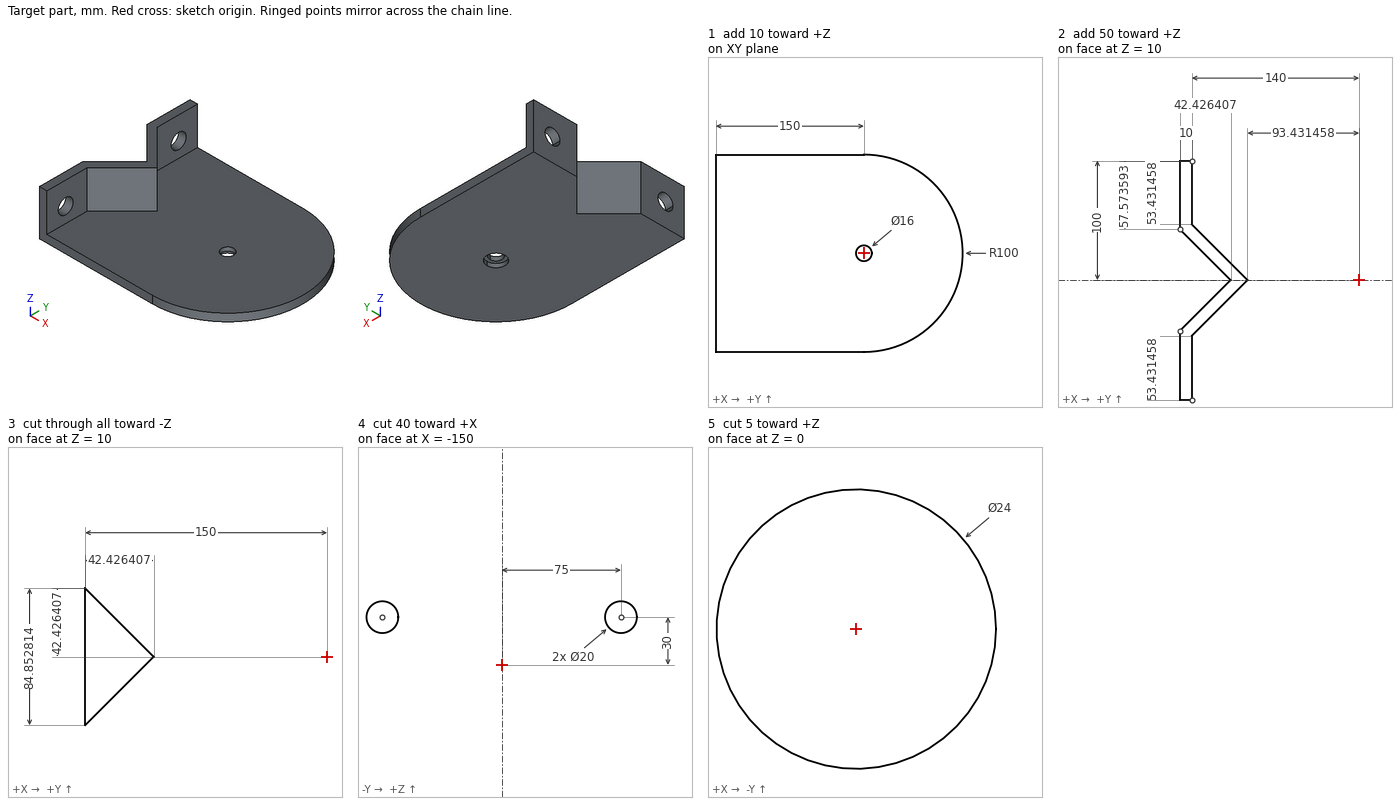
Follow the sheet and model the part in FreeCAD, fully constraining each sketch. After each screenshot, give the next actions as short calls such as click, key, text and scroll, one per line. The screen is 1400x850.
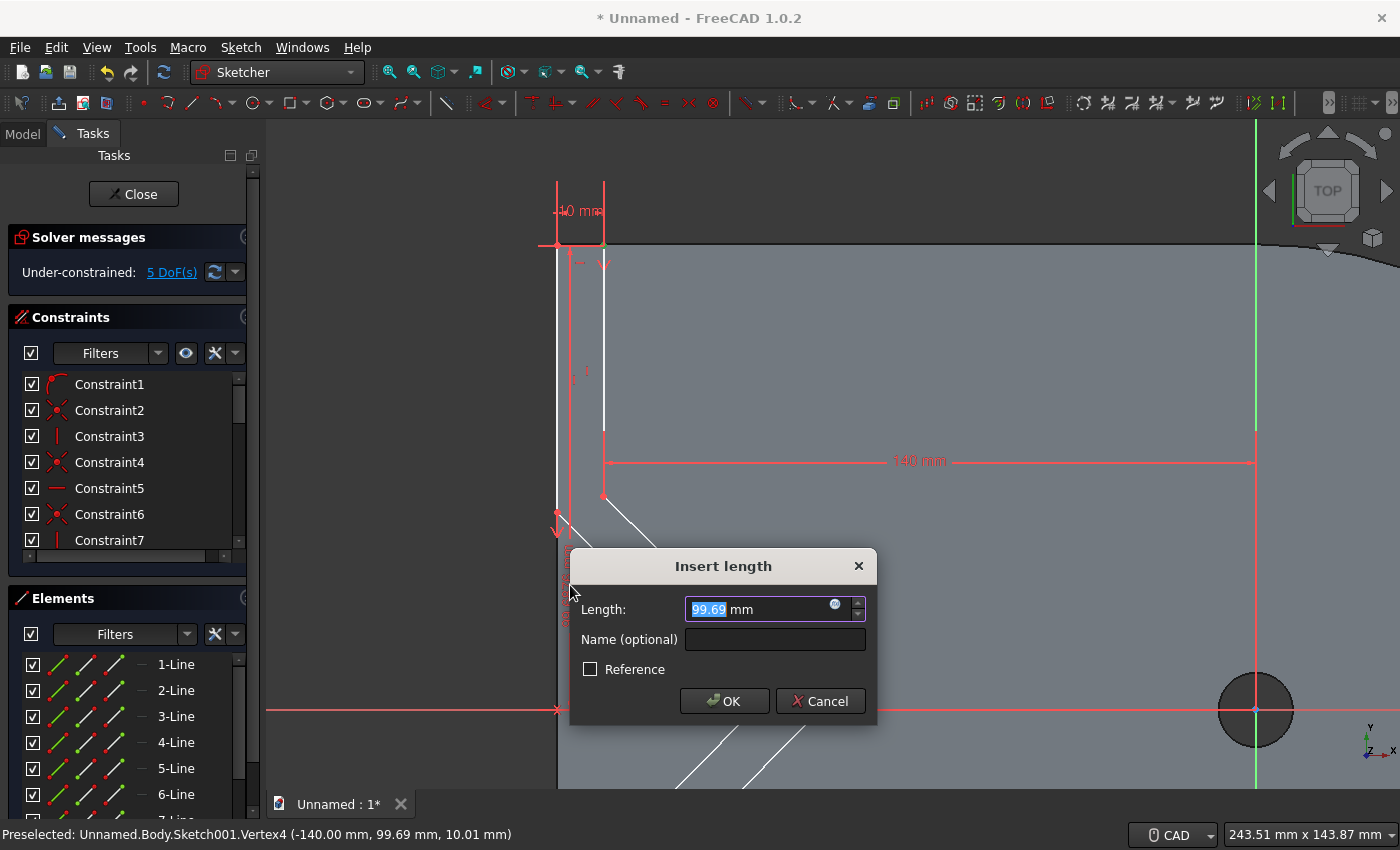
text(100)
key(Return)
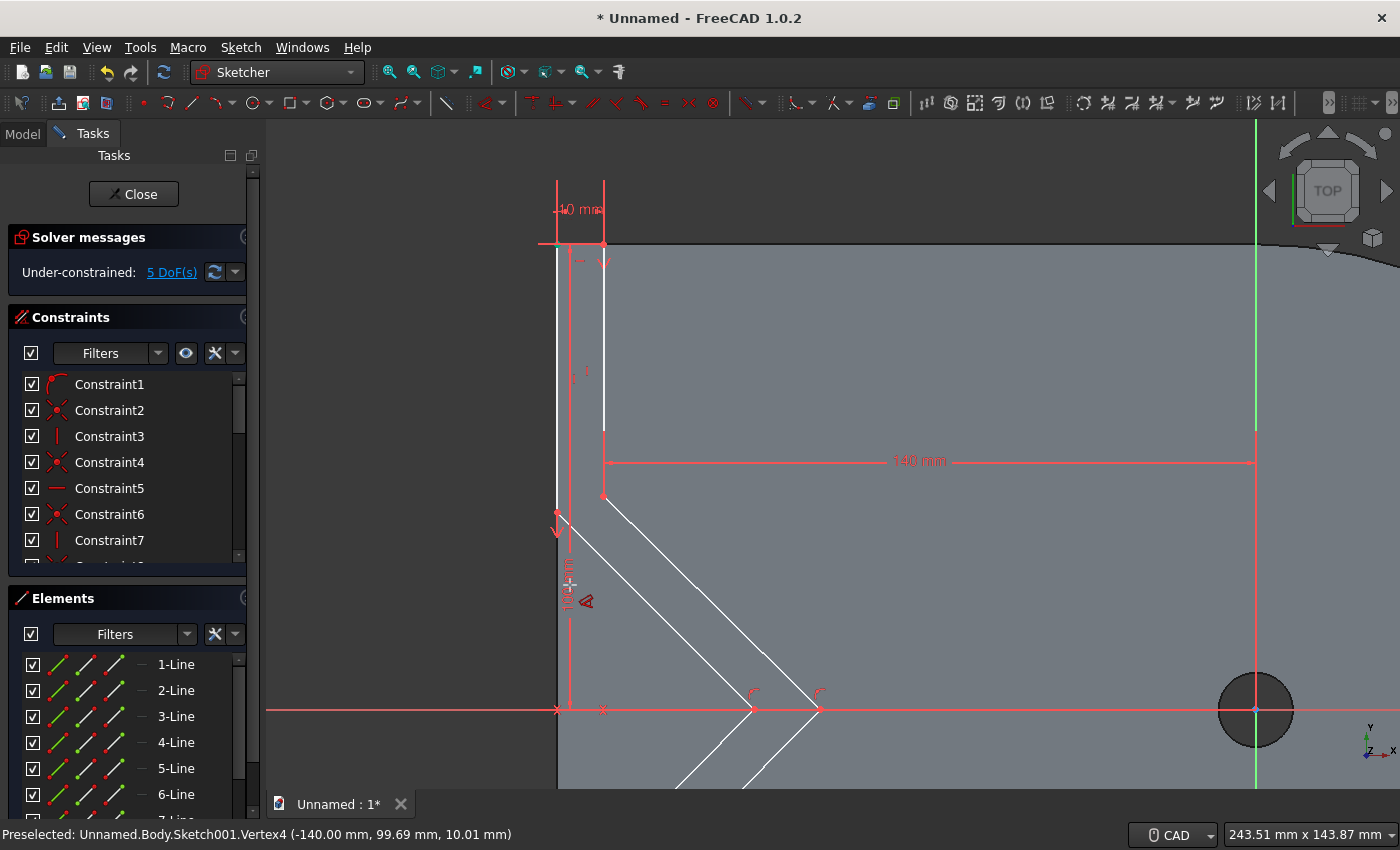
click(604, 421)
click(638, 370)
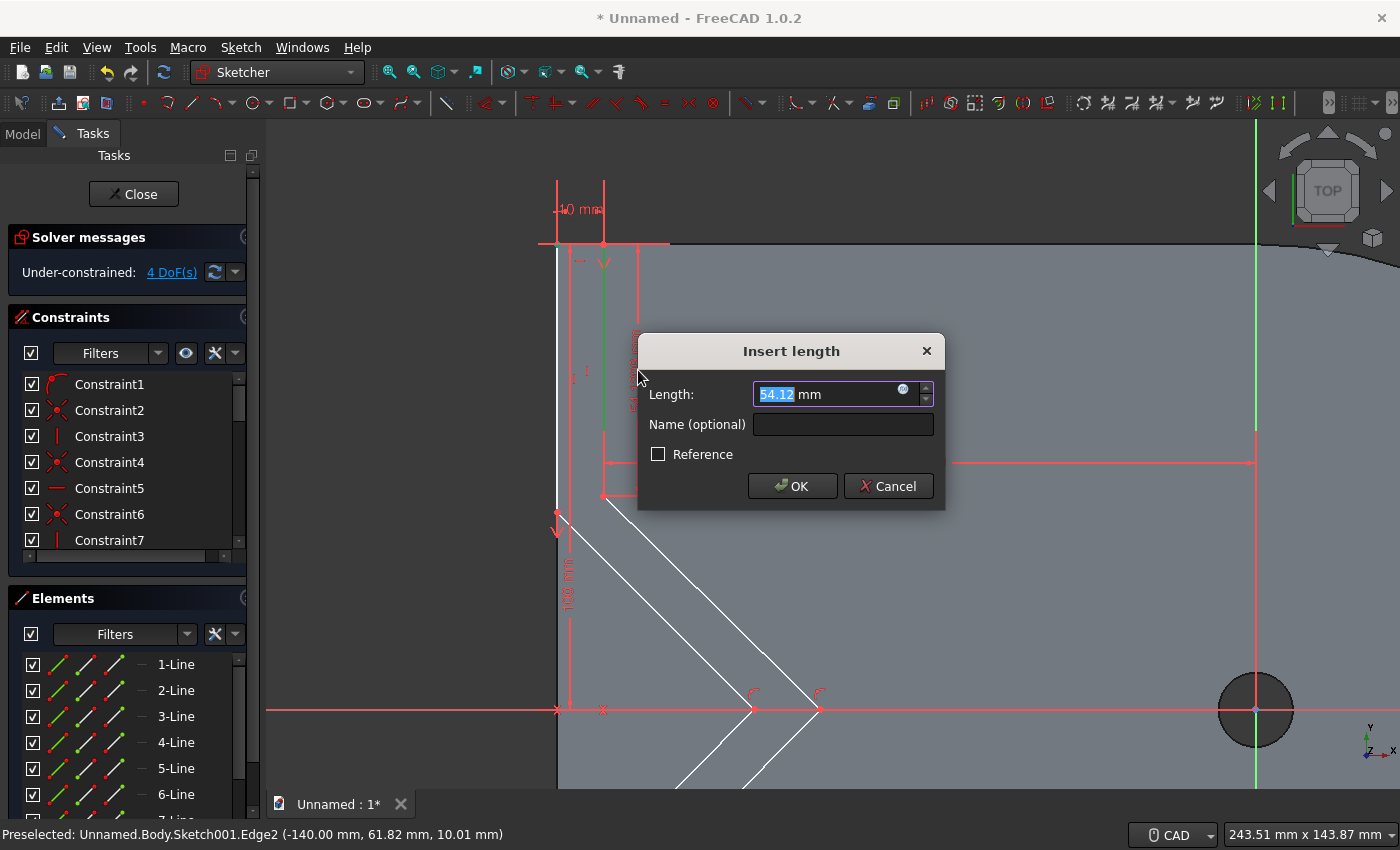
text(53.431458)
key(Return)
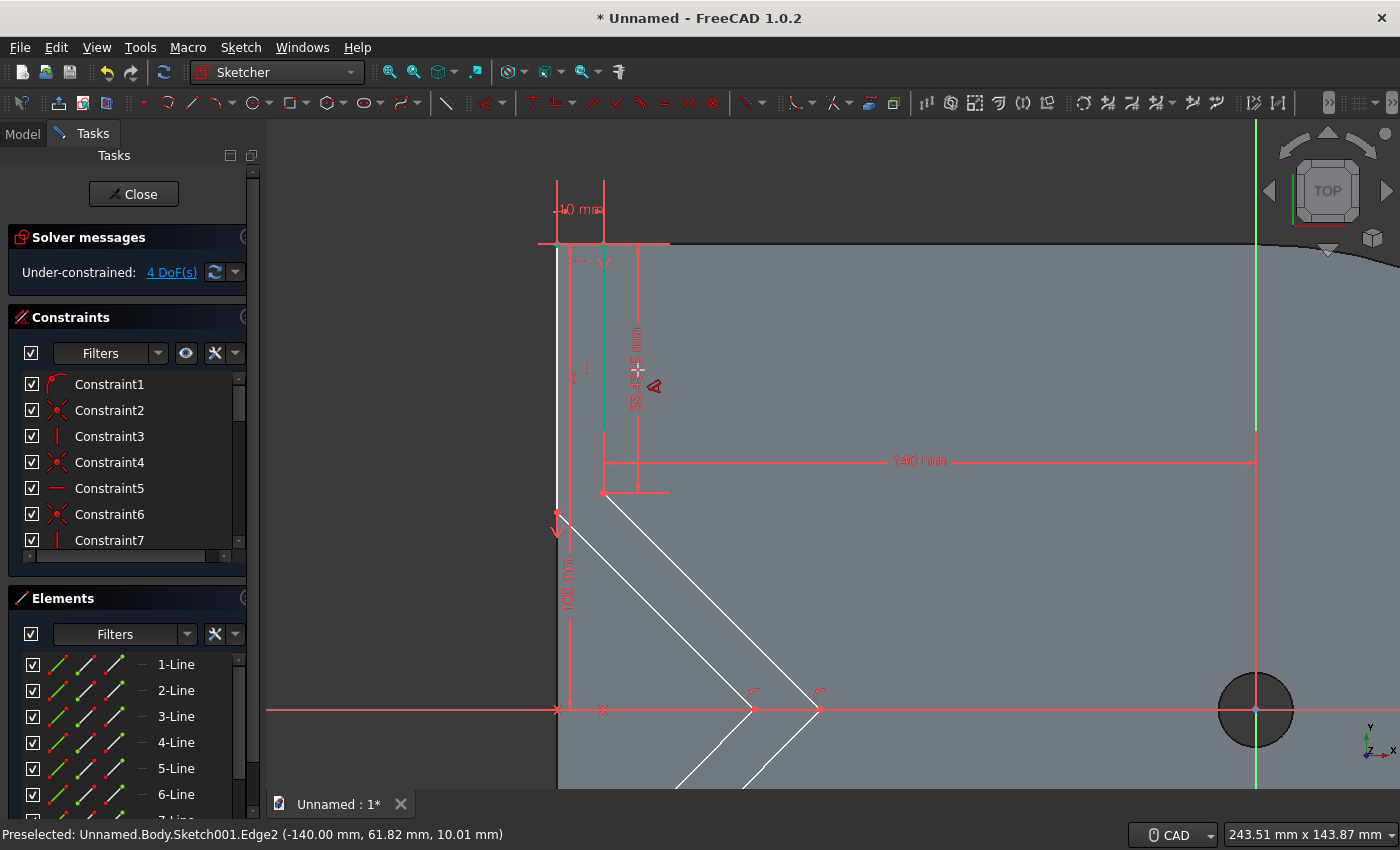
click(557, 325)
click(523, 378)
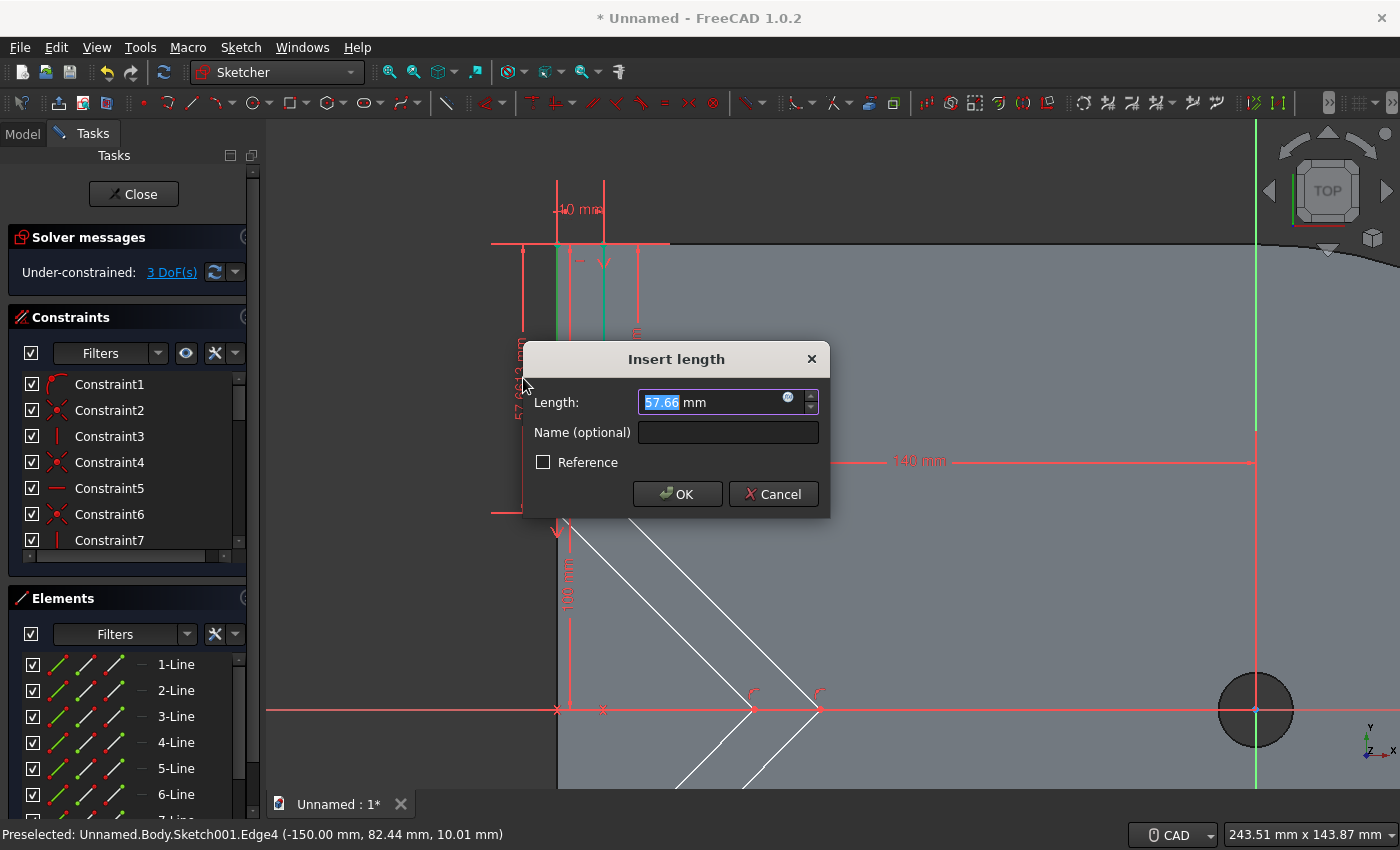
text(57.573593)
key(Return)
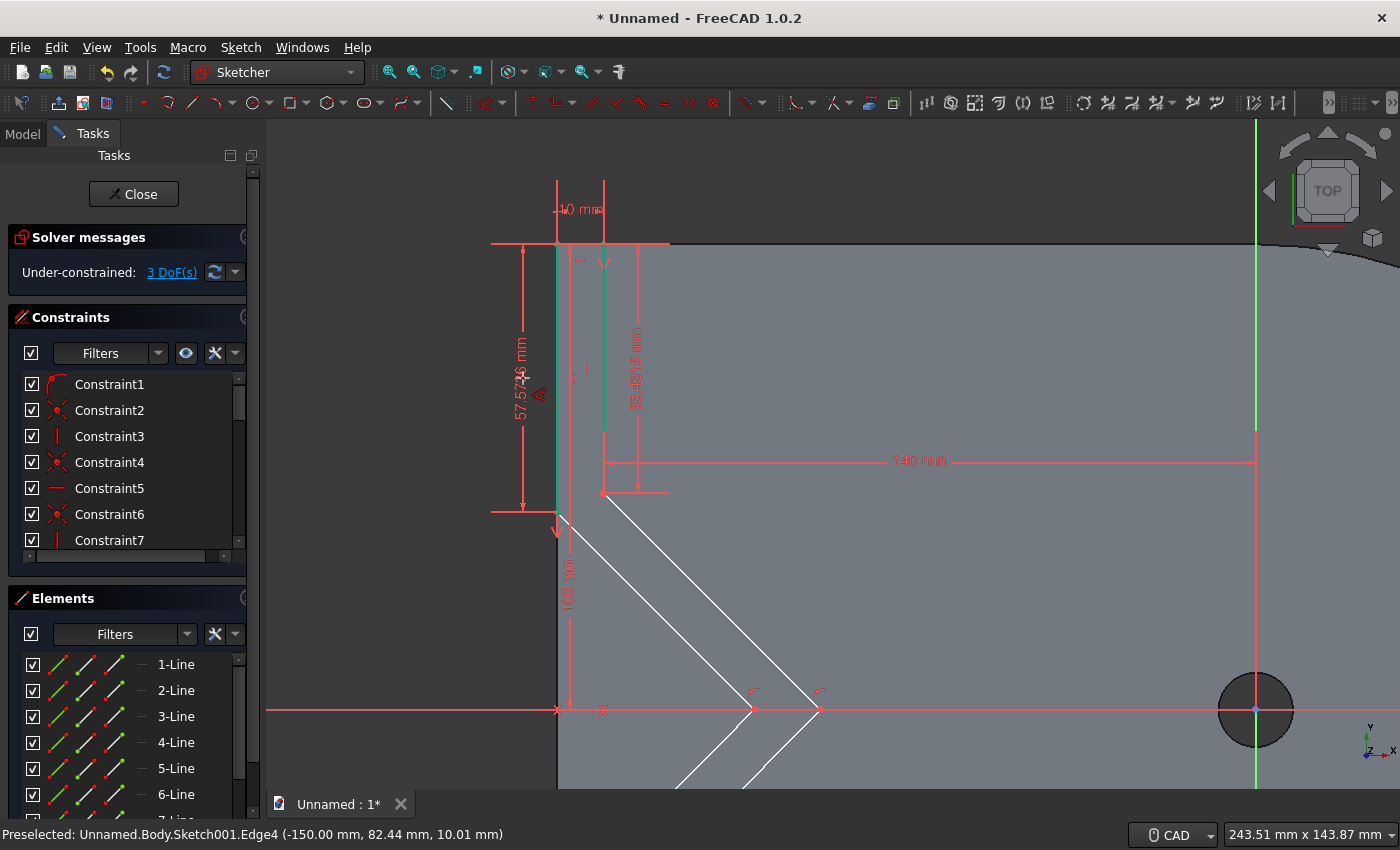
scroll(649, 245, down, 4)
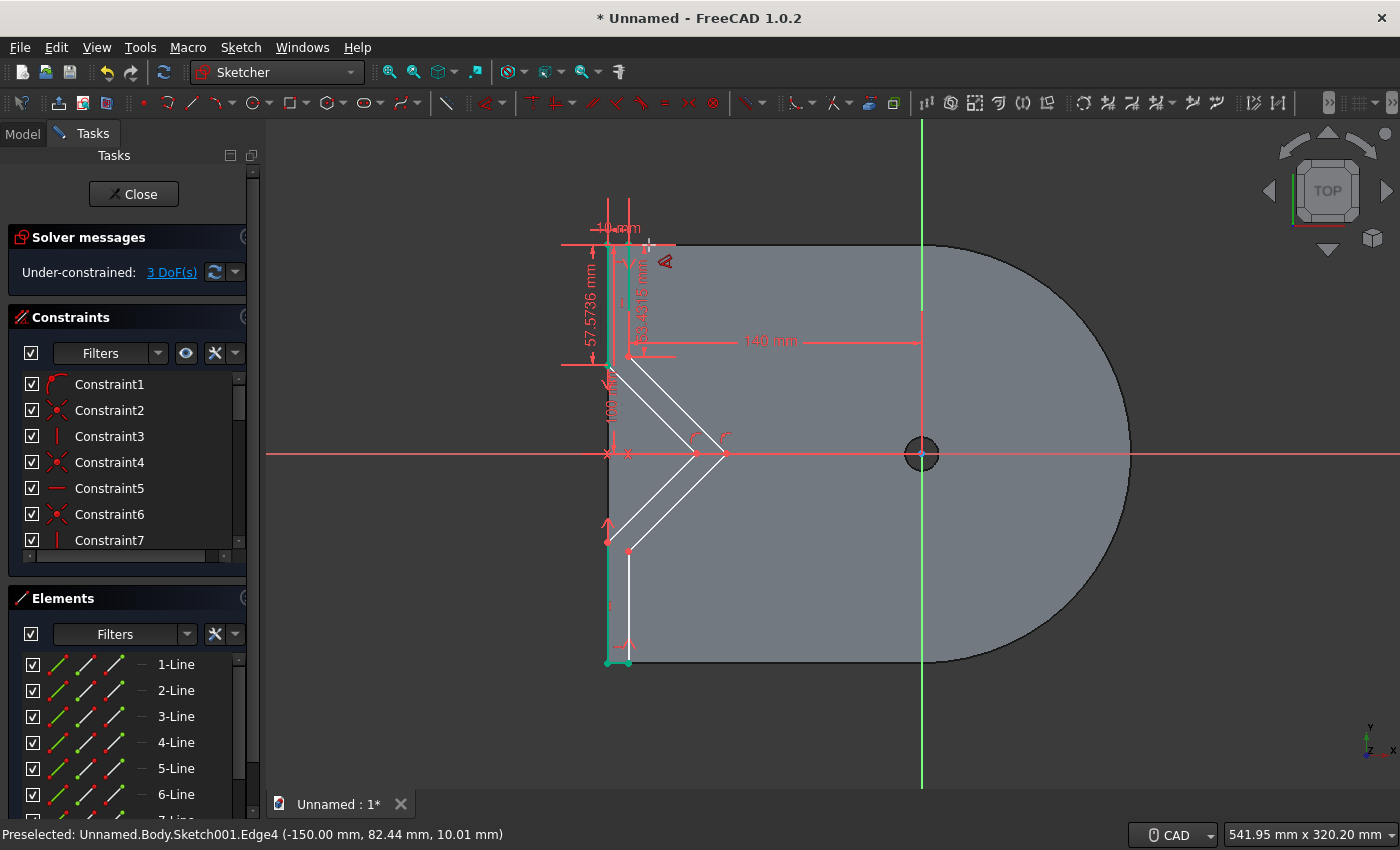
click(629, 630)
click(595, 608)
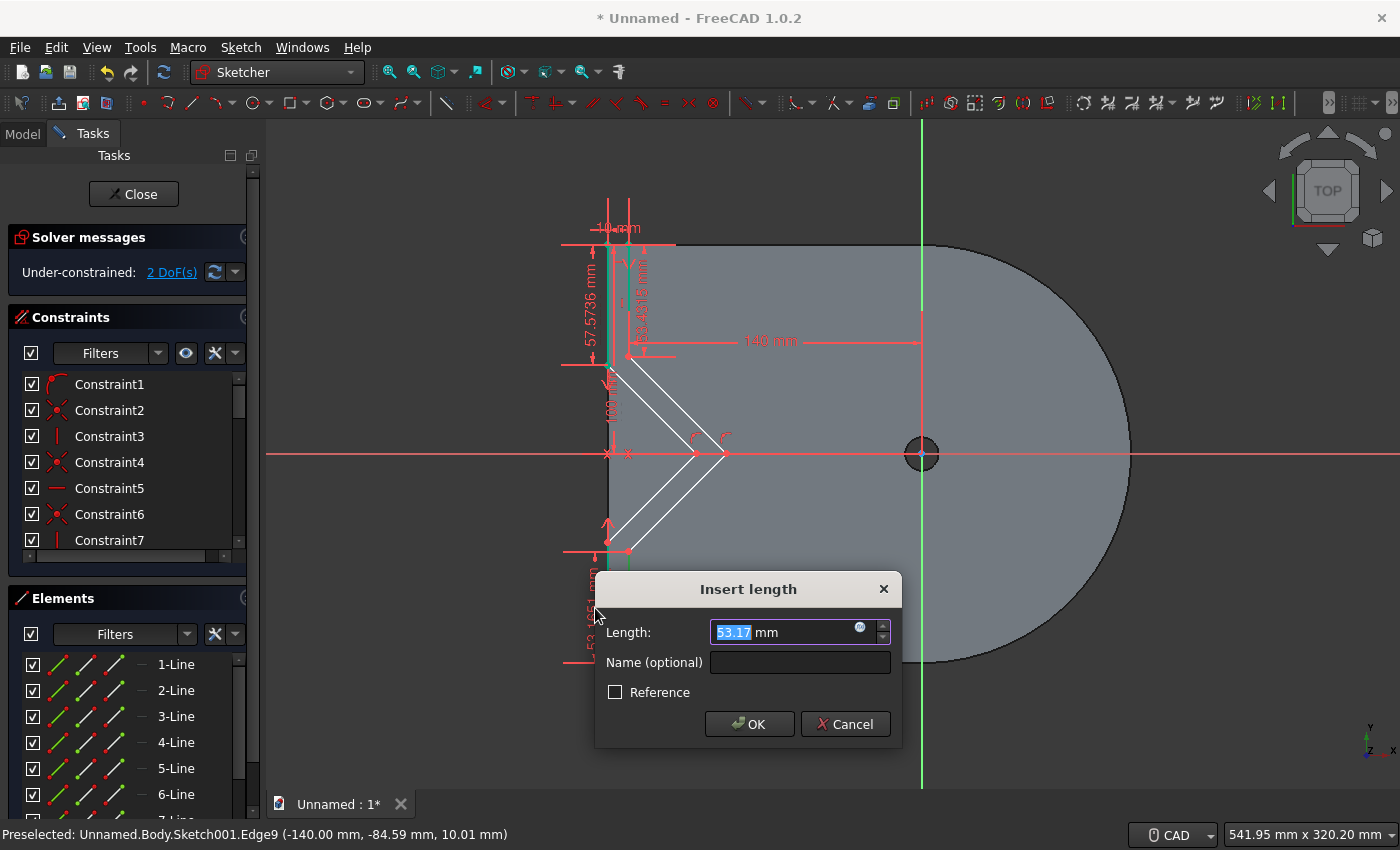
text(53.431458)
key(Return)